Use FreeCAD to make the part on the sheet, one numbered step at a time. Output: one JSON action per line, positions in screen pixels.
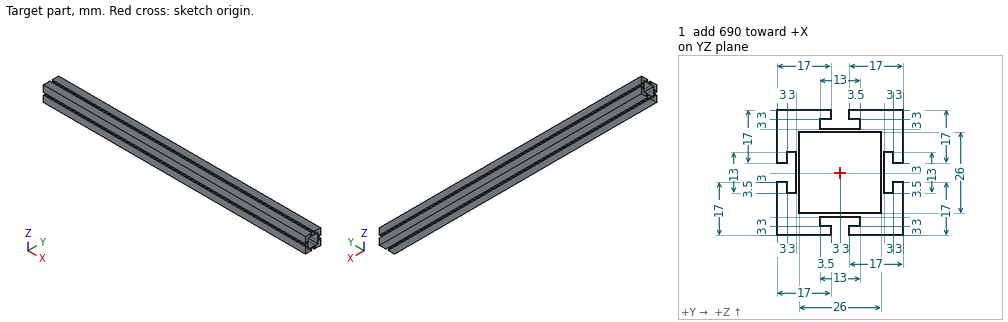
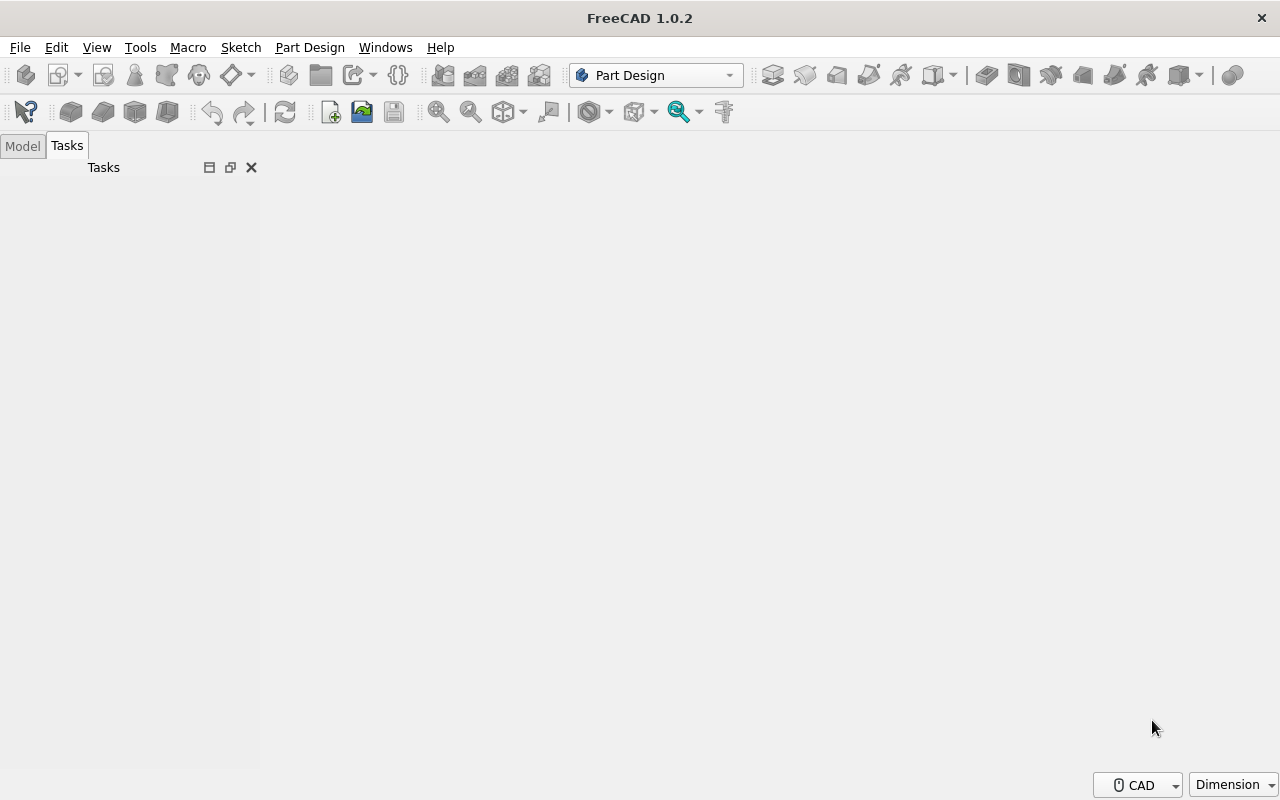
{"action": "key", "text": "ctrl+n"}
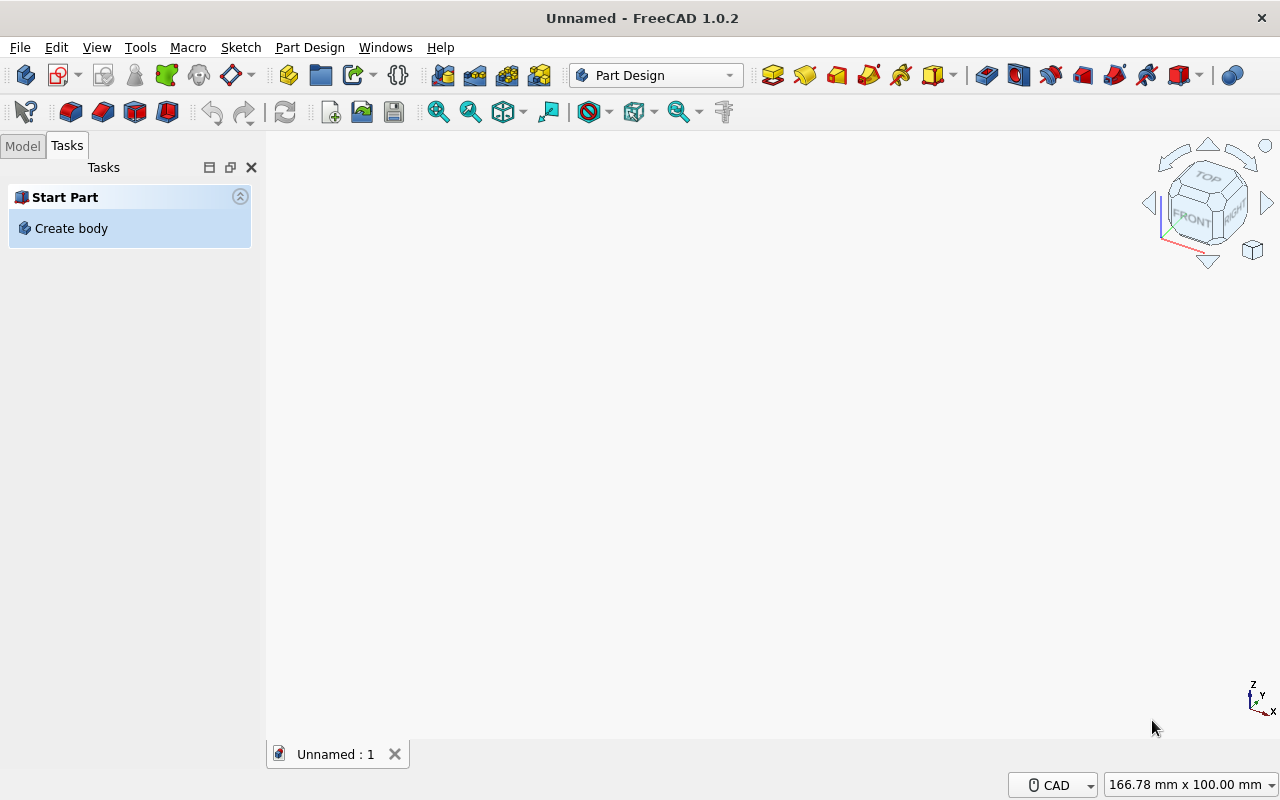
{"action": "left_click", "coordinate": [58, 76]}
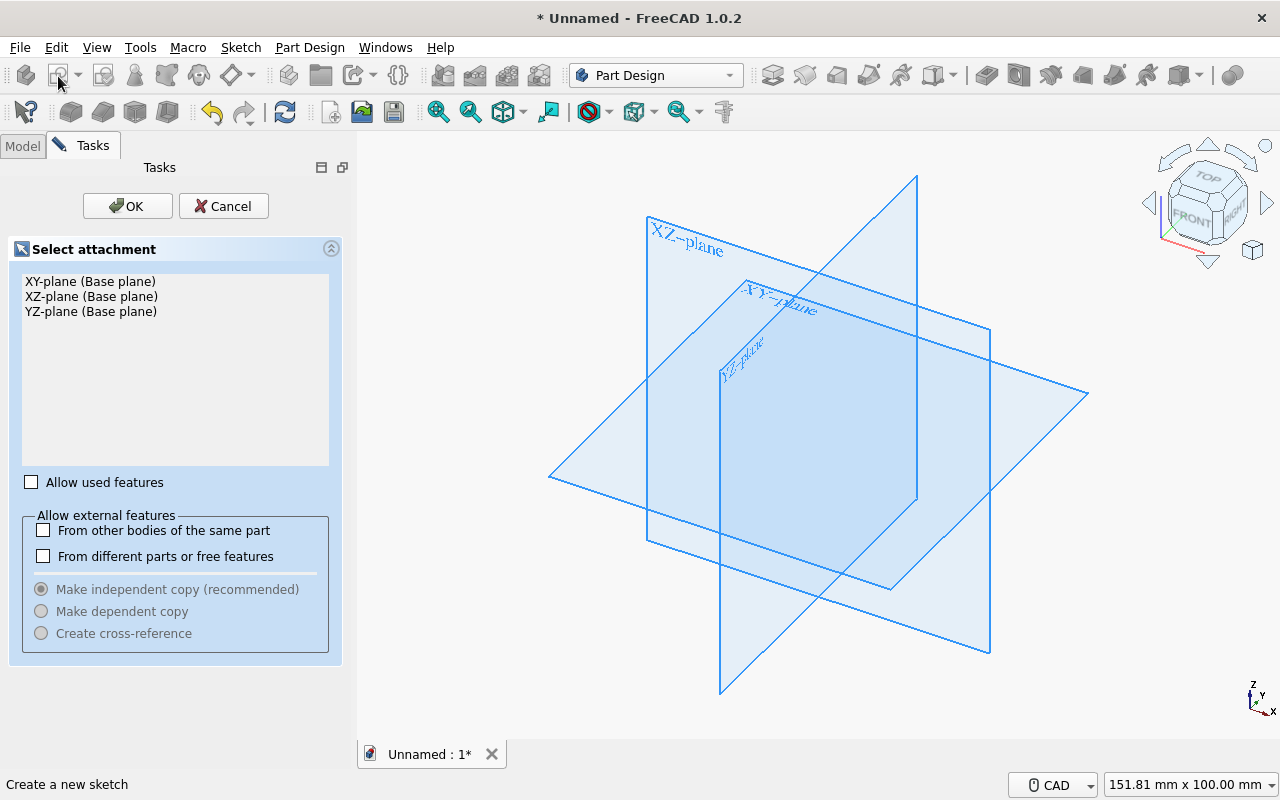
{"action": "left_click", "coordinate": [82, 312]}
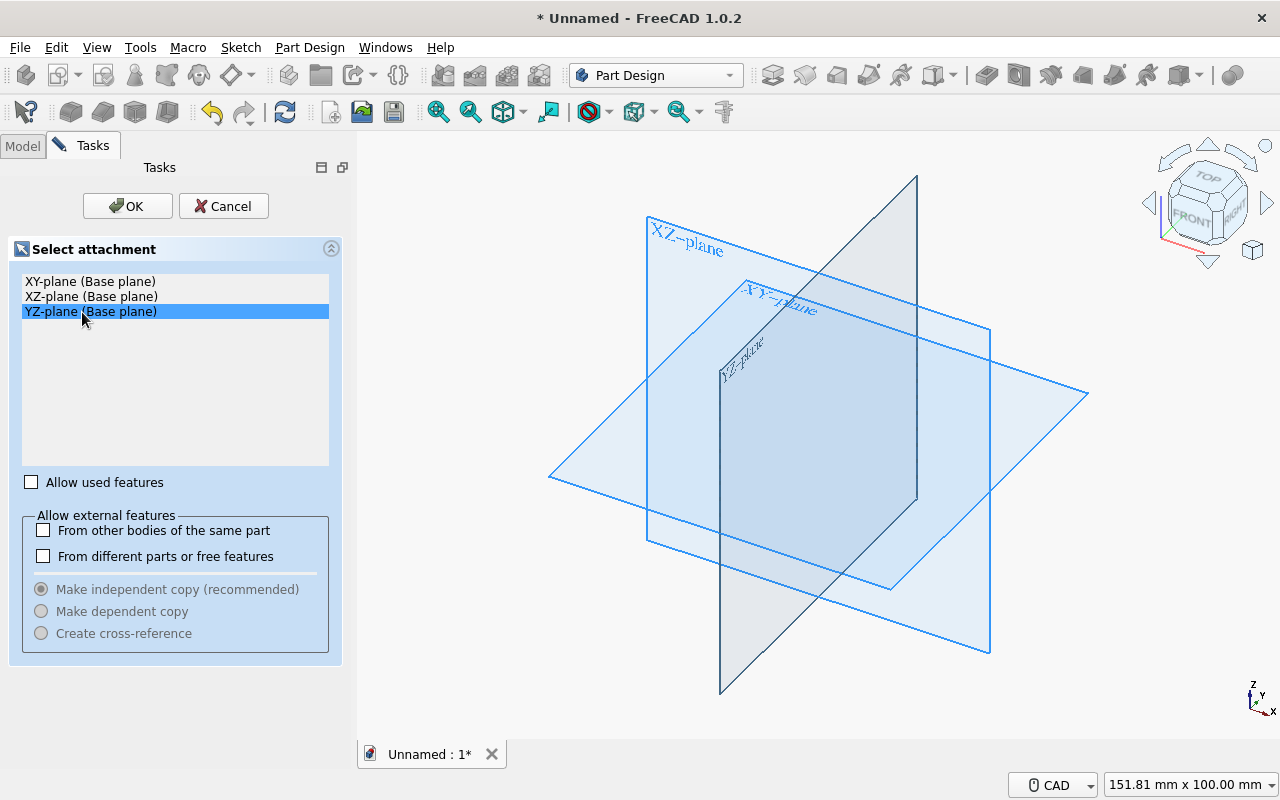
{"action": "left_click", "coordinate": [128, 206]}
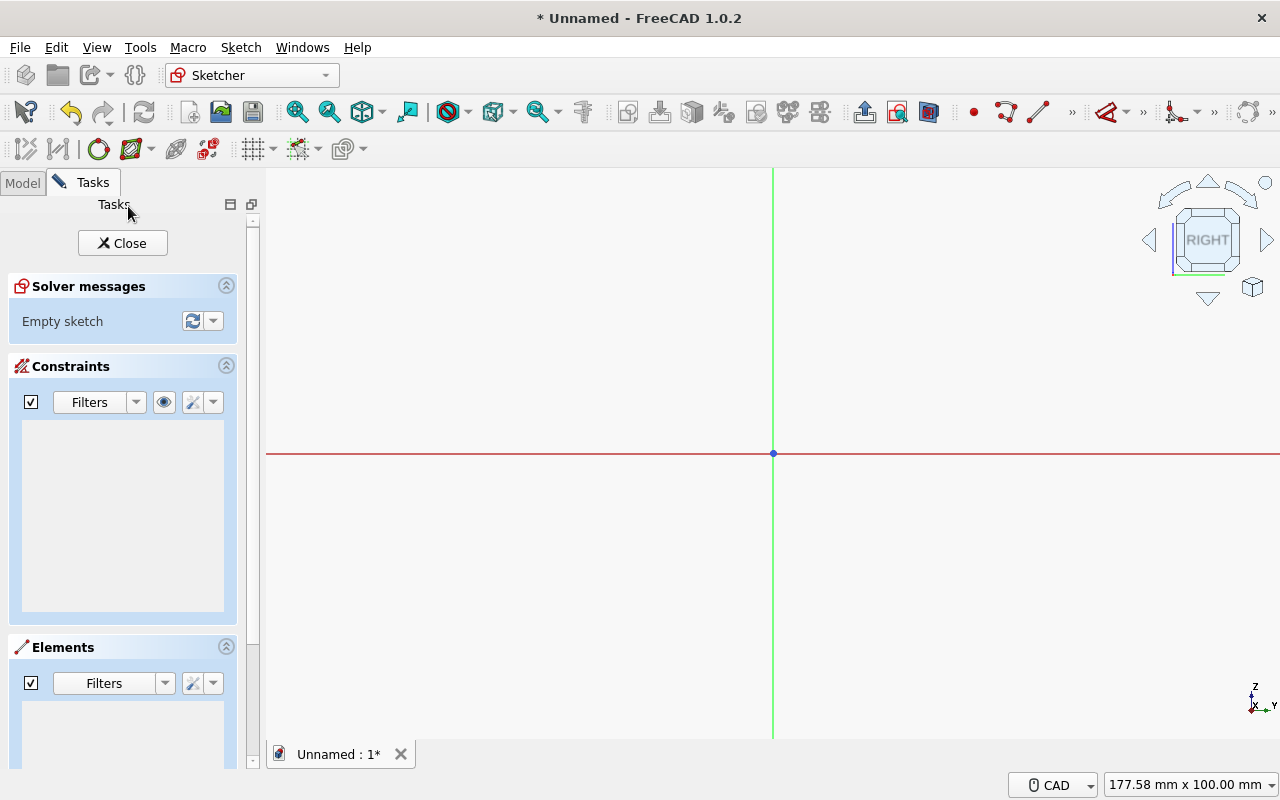
{"action": "scroll", "coordinate": [912, 454], "scroll_direction": "up", "scroll_amount": 2}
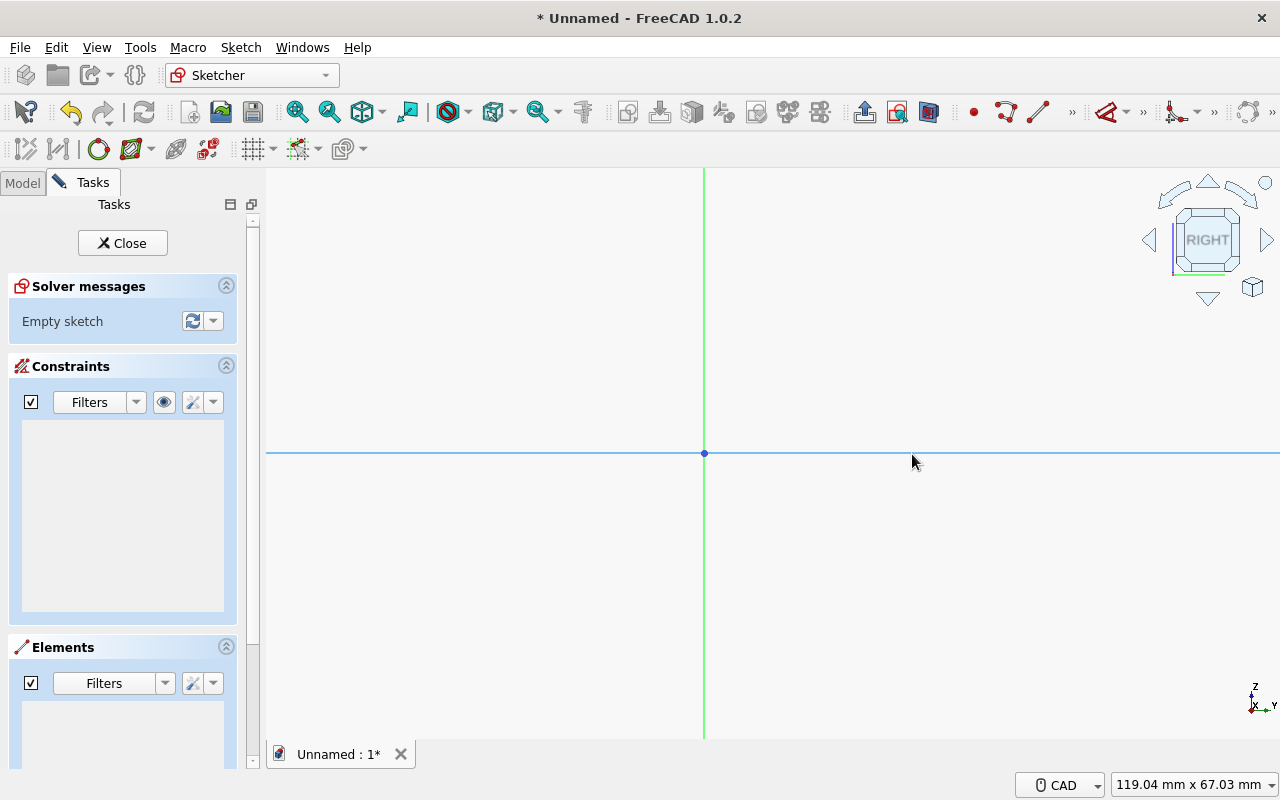
{"action": "key", "text": "g m"}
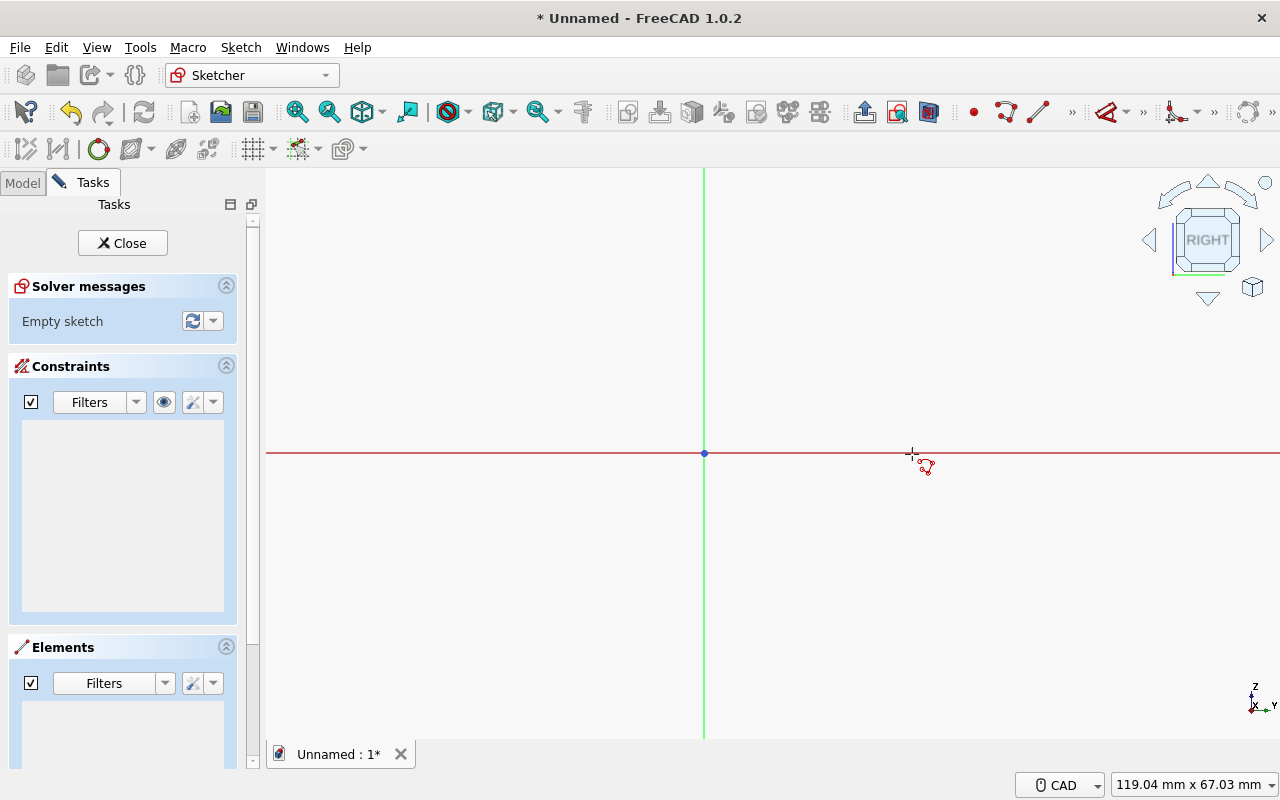
{"action": "left_click", "coordinate": [585, 398]}
{"action": "left_click", "coordinate": [585, 508]}
{"action": "left_click", "coordinate": [560, 508]}
{"action": "left_click", "coordinate": [560, 479]}
{"action": "left_click", "coordinate": [534, 479]}
{"action": "left_click", "coordinate": [534, 623]}
{"action": "left_click", "coordinate": [679, 623]}
{"action": "left_click", "coordinate": [679, 598]}
{"action": "left_click", "coordinate": [649, 598]}
{"action": "left_click", "coordinate": [649, 572]}
{"action": "left_click", "coordinate": [760, 572]}
{"action": "left_click", "coordinate": [760, 598]}
{"action": "left_click", "coordinate": [730, 598]}
{"action": "left_click", "coordinate": [730, 623]}
{"action": "left_click", "coordinate": [875, 623]}
{"action": "left_click", "coordinate": [875, 479]}
{"action": "left_click", "coordinate": [849, 479]}
{"action": "left_click", "coordinate": [849, 508]}
{"action": "left_click", "coordinate": [824, 508]}
{"action": "left_click", "coordinate": [824, 398]}
{"action": "left_click", "coordinate": [849, 398]}
{"action": "left_click", "coordinate": [849, 427]}
{"action": "left_click", "coordinate": [875, 427]}
{"action": "left_click", "coordinate": [875, 283]}
{"action": "left_click", "coordinate": [730, 283]}
{"action": "left_click", "coordinate": [730, 308]}
{"action": "left_click", "coordinate": [760, 308]}
{"action": "left_click", "coordinate": [760, 334]}
{"action": "left_click", "coordinate": [649, 334]}
{"action": "left_click", "coordinate": [649, 308]}
{"action": "left_click", "coordinate": [679, 308]}
{"action": "left_click", "coordinate": [679, 283]}
{"action": "left_click", "coordinate": [534, 283]}
{"action": "left_click", "coordinate": [534, 427]}
{"action": "left_click", "coordinate": [560, 427]}
{"action": "left_click", "coordinate": [560, 398]}
{"action": "left_click", "coordinate": [585, 399]}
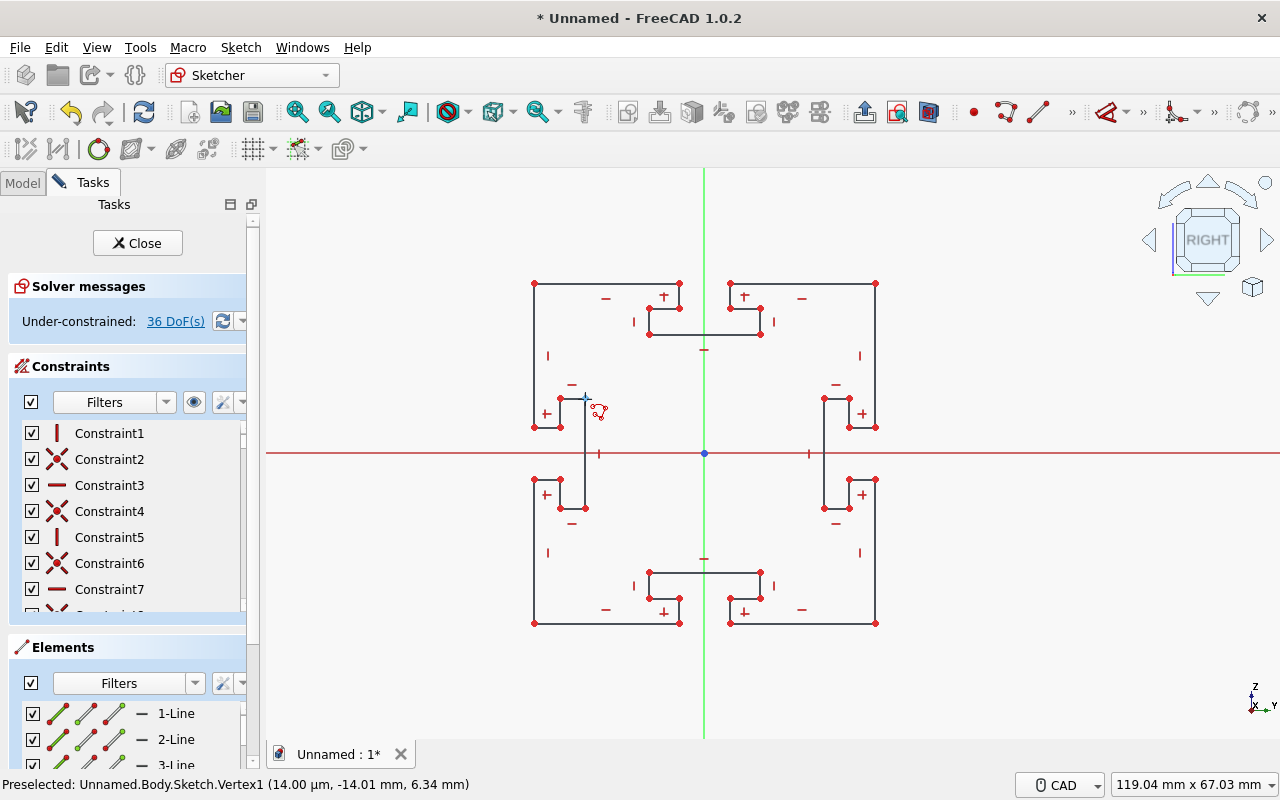
{"action": "key", "text": "g v"}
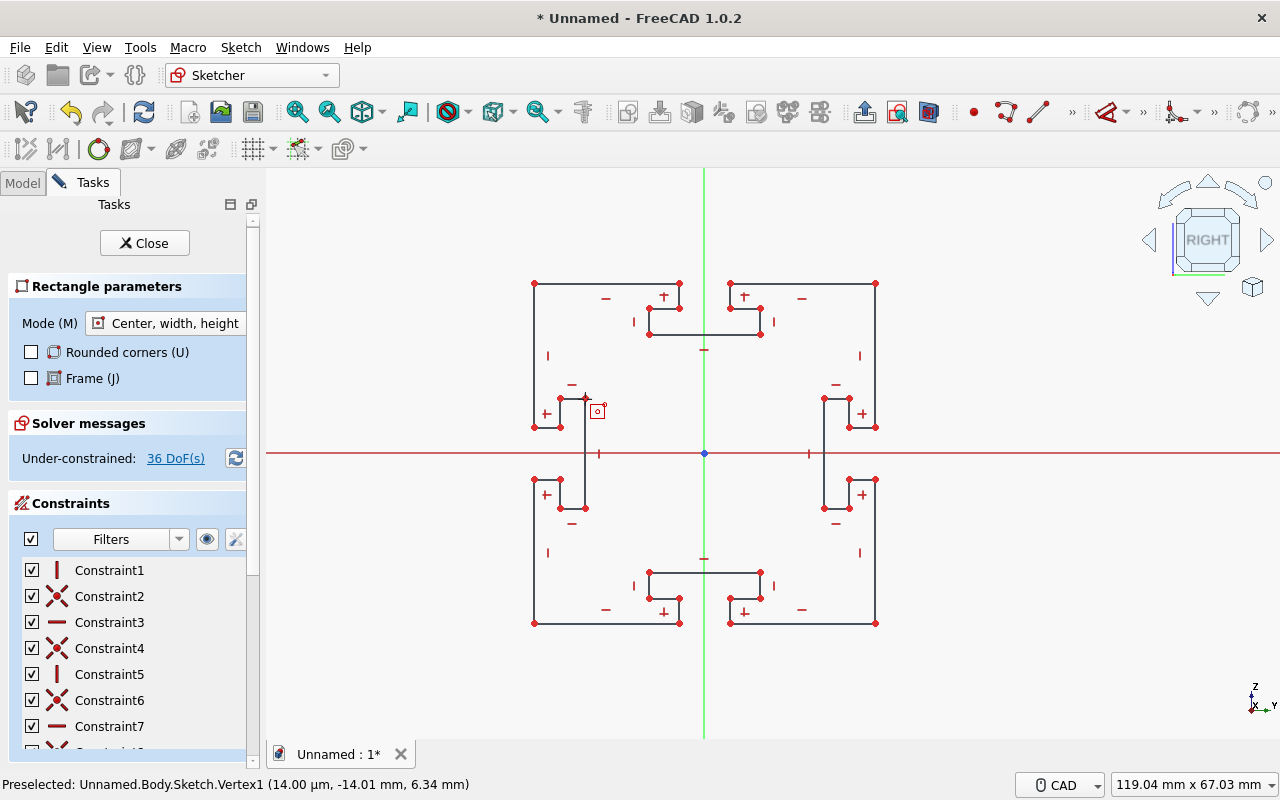
{"action": "left_click", "coordinate": [704, 453]}
{"action": "mouse_move", "coordinate": [815, 342]}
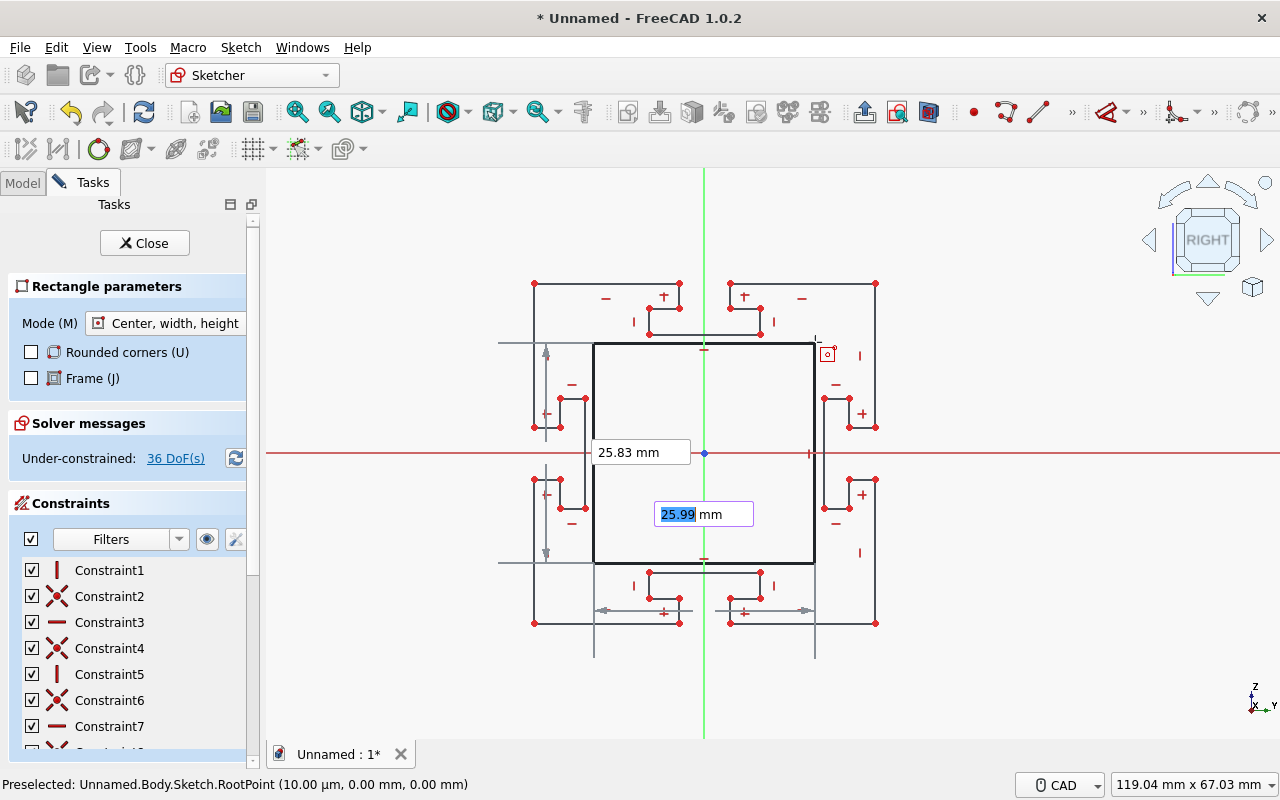
{"action": "type", "text": "26"}
{"action": "key", "text": "Tab"}
{"action": "type", "text": "26"}
{"action": "key", "text": "Return"}
{"action": "key", "text": "Escape"}